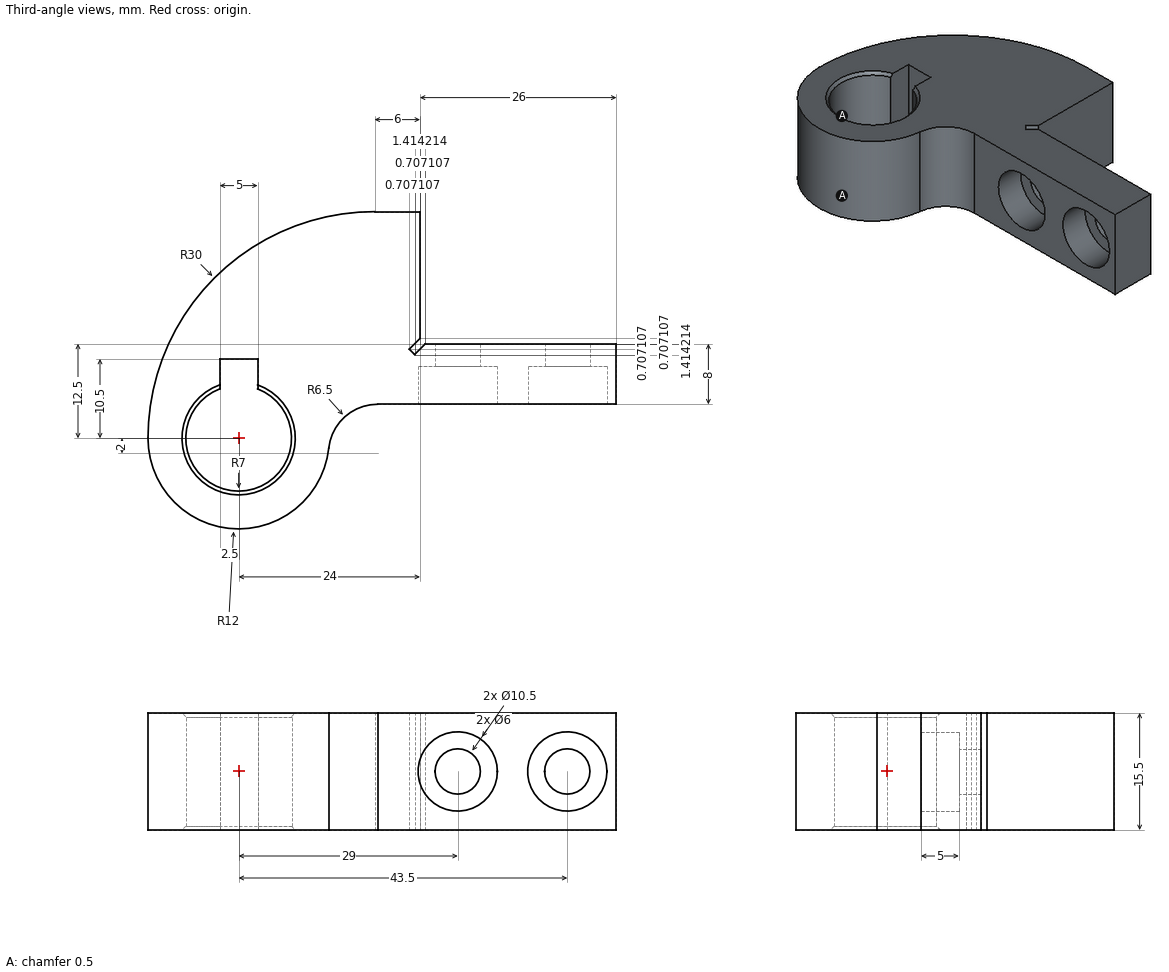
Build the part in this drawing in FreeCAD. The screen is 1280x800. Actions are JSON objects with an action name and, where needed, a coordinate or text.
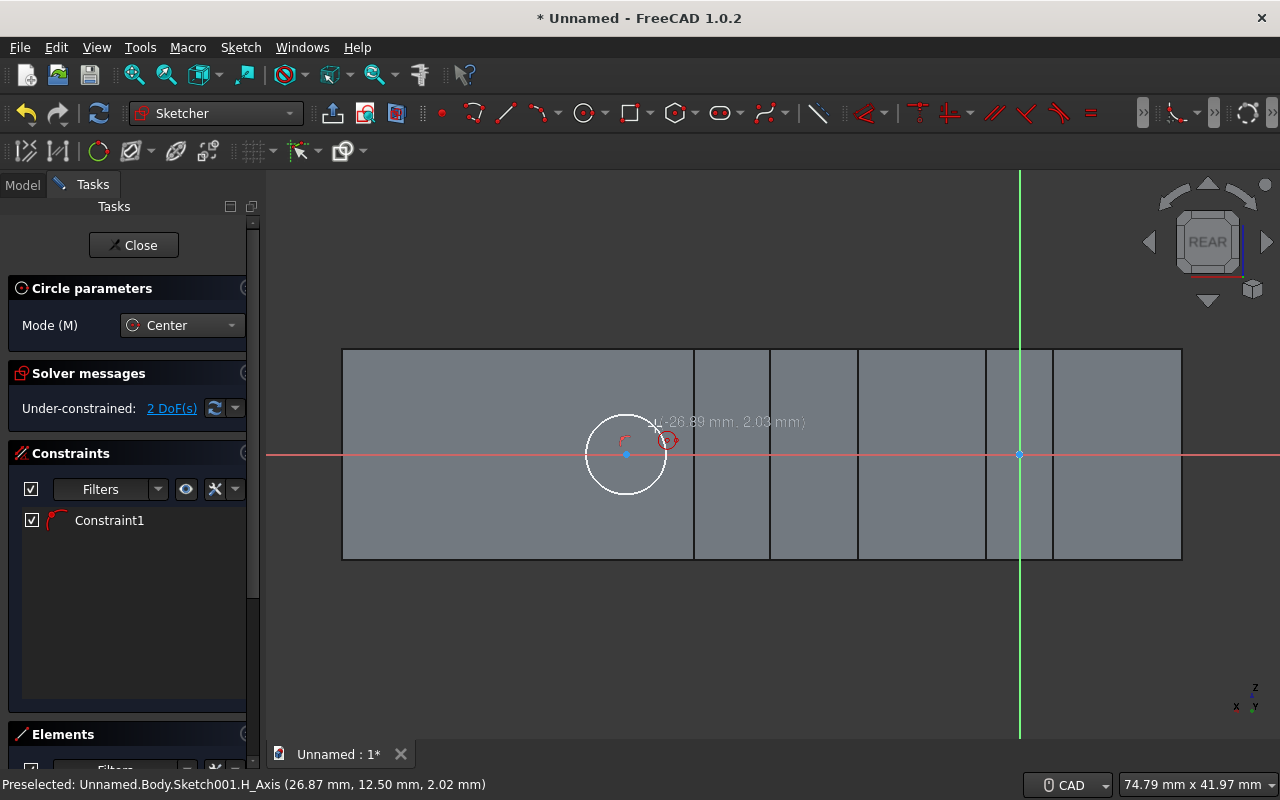
{"action": "left_click", "coordinate": [430, 454]}
{"action": "left_click", "coordinate": [459, 426]}
{"action": "key", "text": "Escape"}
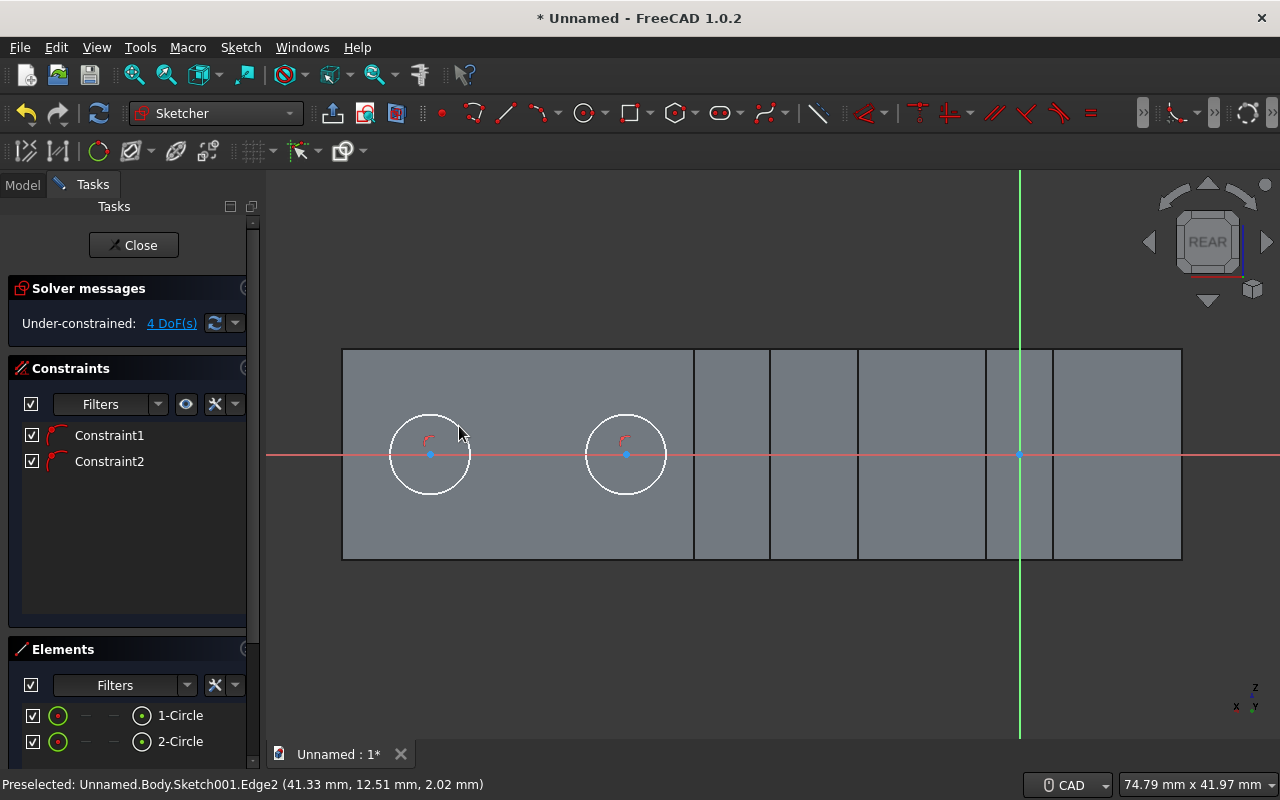
{"action": "left_click", "coordinate": [654, 426]}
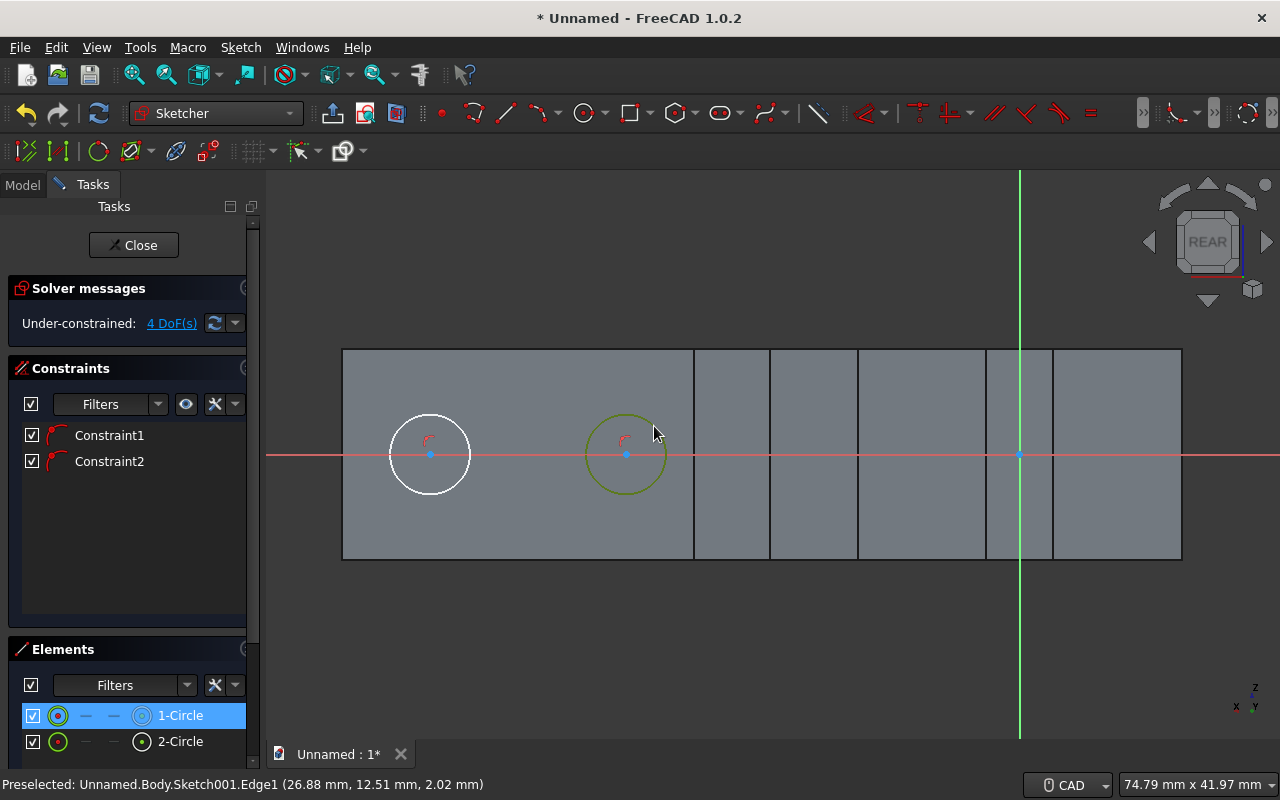
{"action": "left_click", "coordinate": [458, 426]}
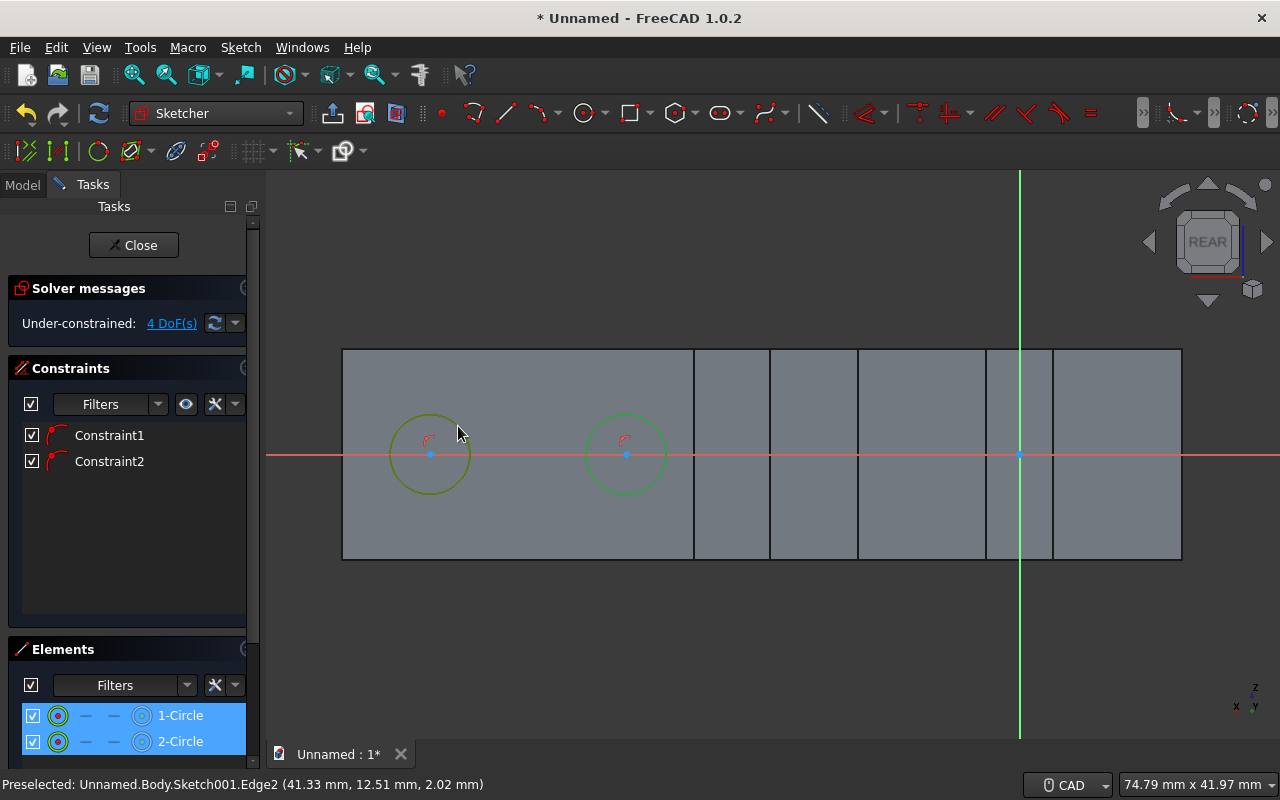
{"action": "left_click", "coordinate": [1092, 114]}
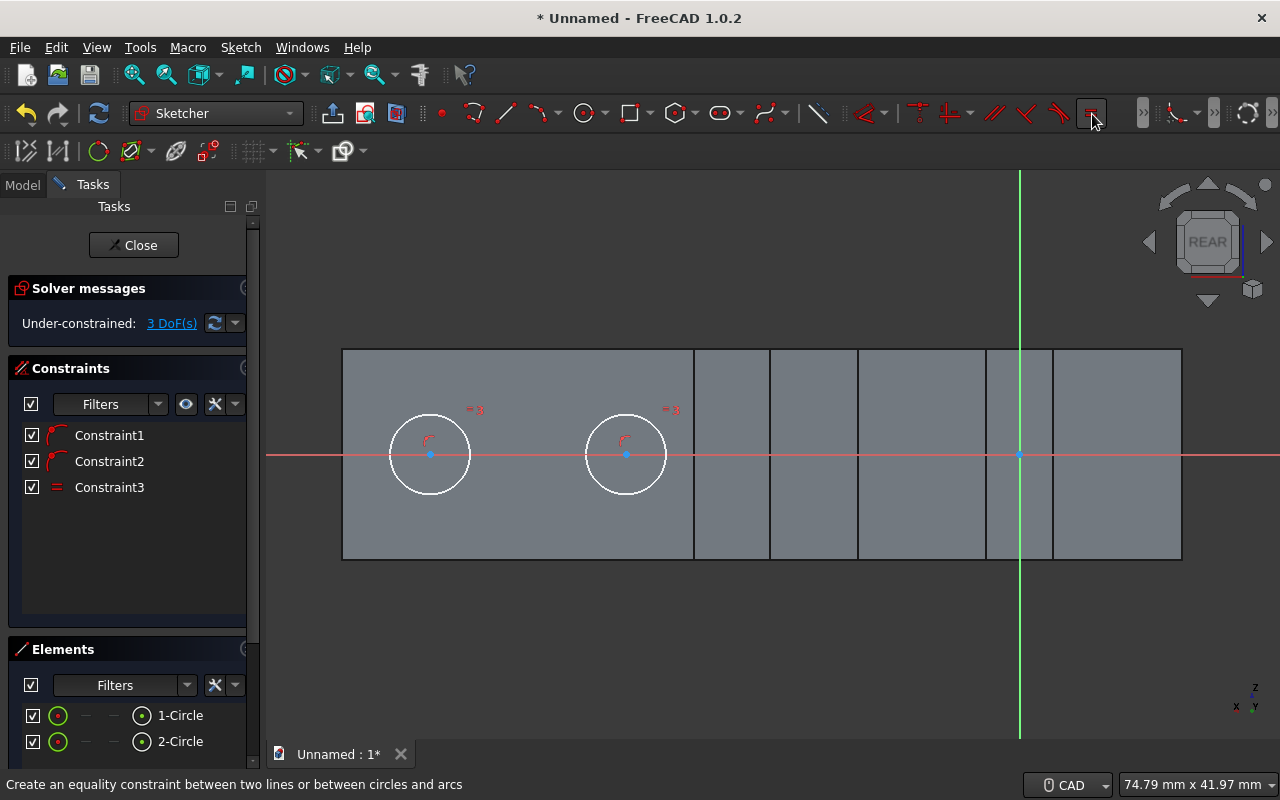
{"action": "left_click", "coordinate": [864, 114]}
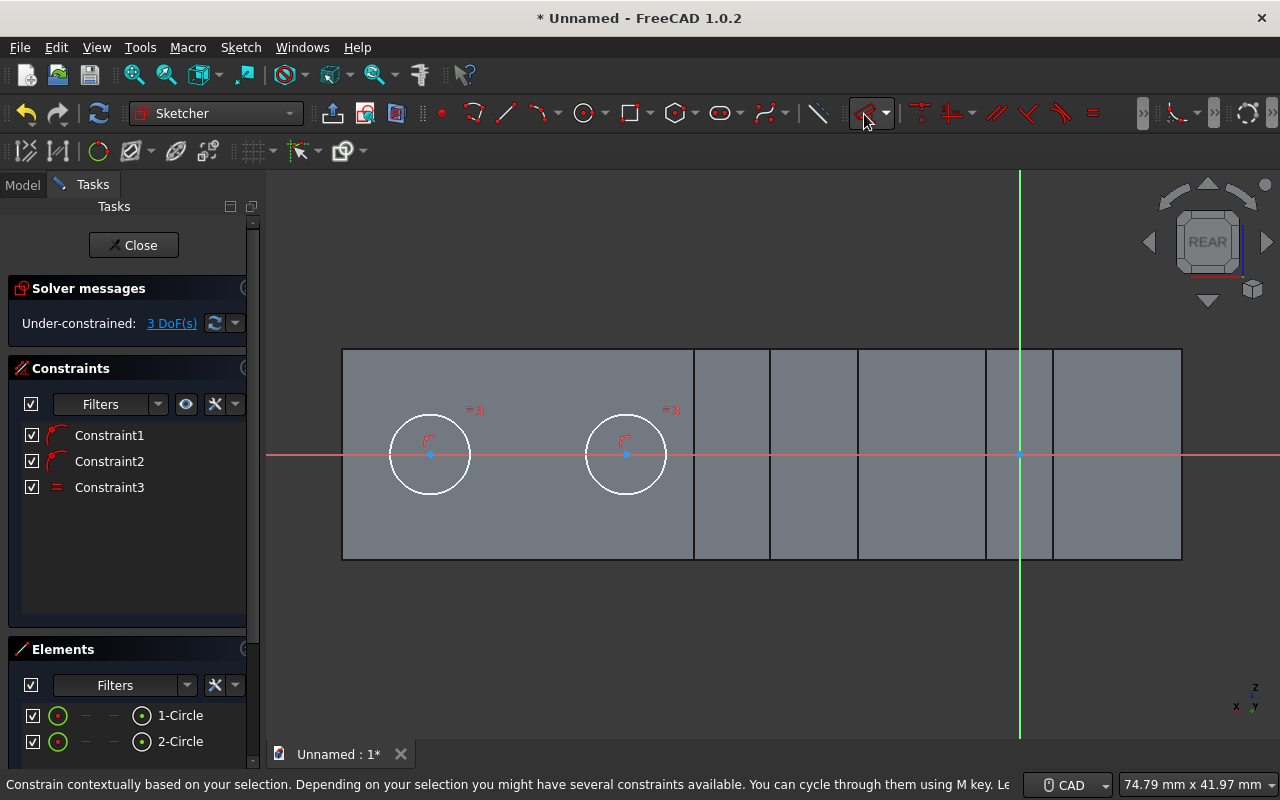
{"action": "left_click", "coordinate": [654, 426]}
{"action": "left_click", "coordinate": [676, 403]}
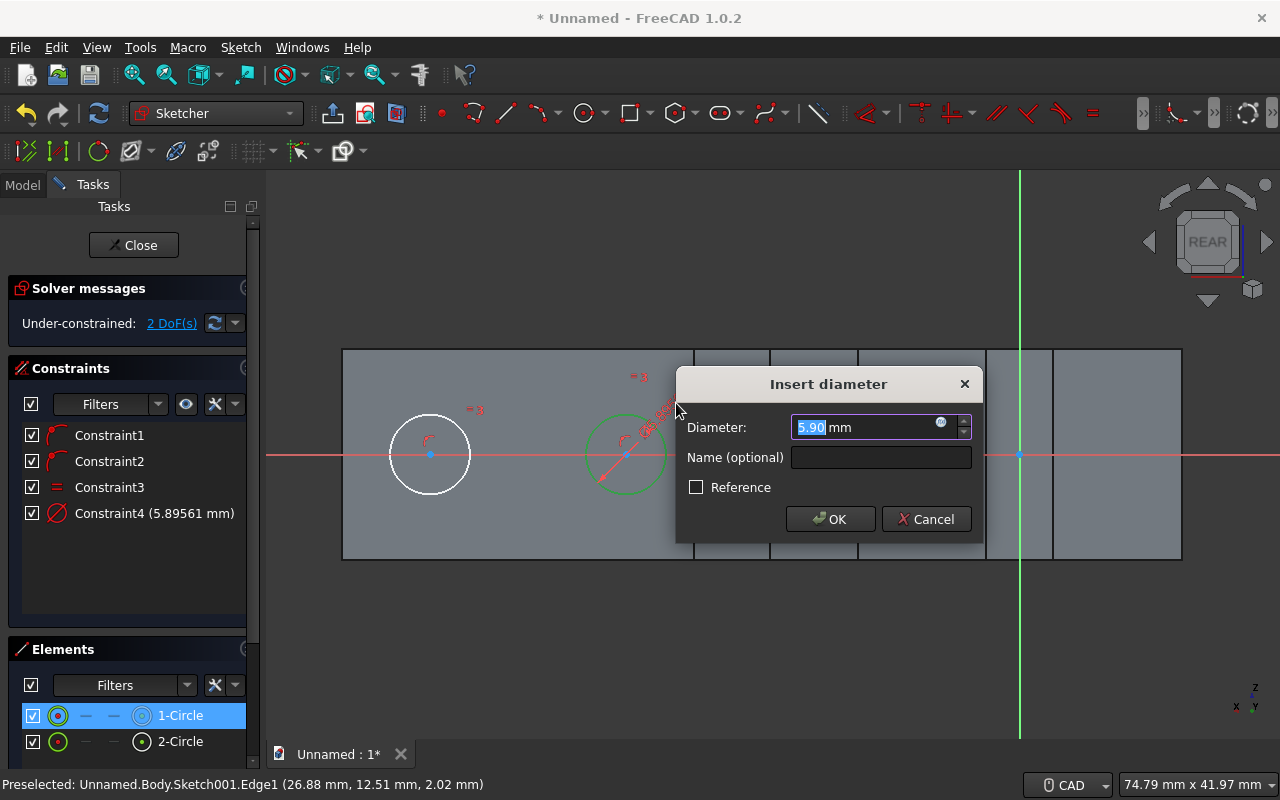
{"action": "type", "text": "6"}
{"action": "key", "text": "Return"}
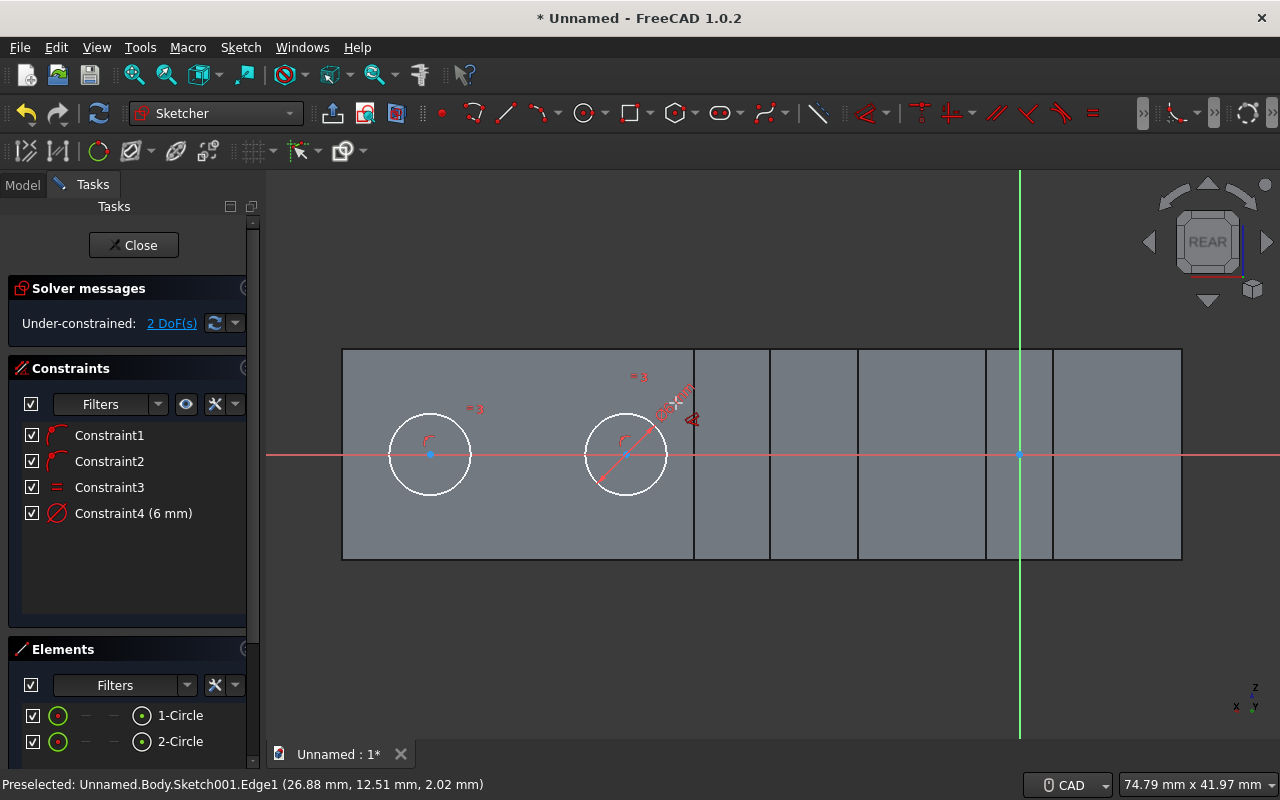
{"action": "left_click", "coordinate": [626, 454]}
{"action": "left_click", "coordinate": [823, 488]}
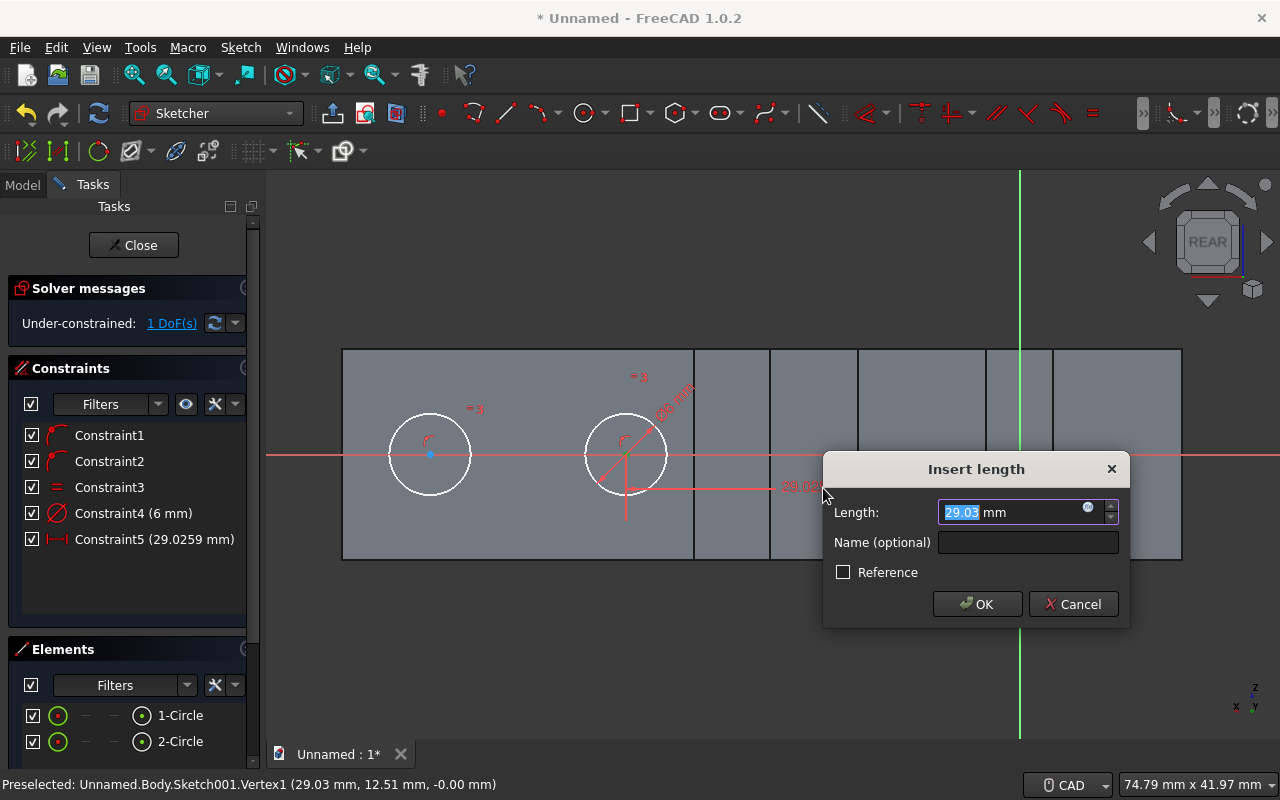
{"action": "type", "text": "29"}
{"action": "key", "text": "Return"}